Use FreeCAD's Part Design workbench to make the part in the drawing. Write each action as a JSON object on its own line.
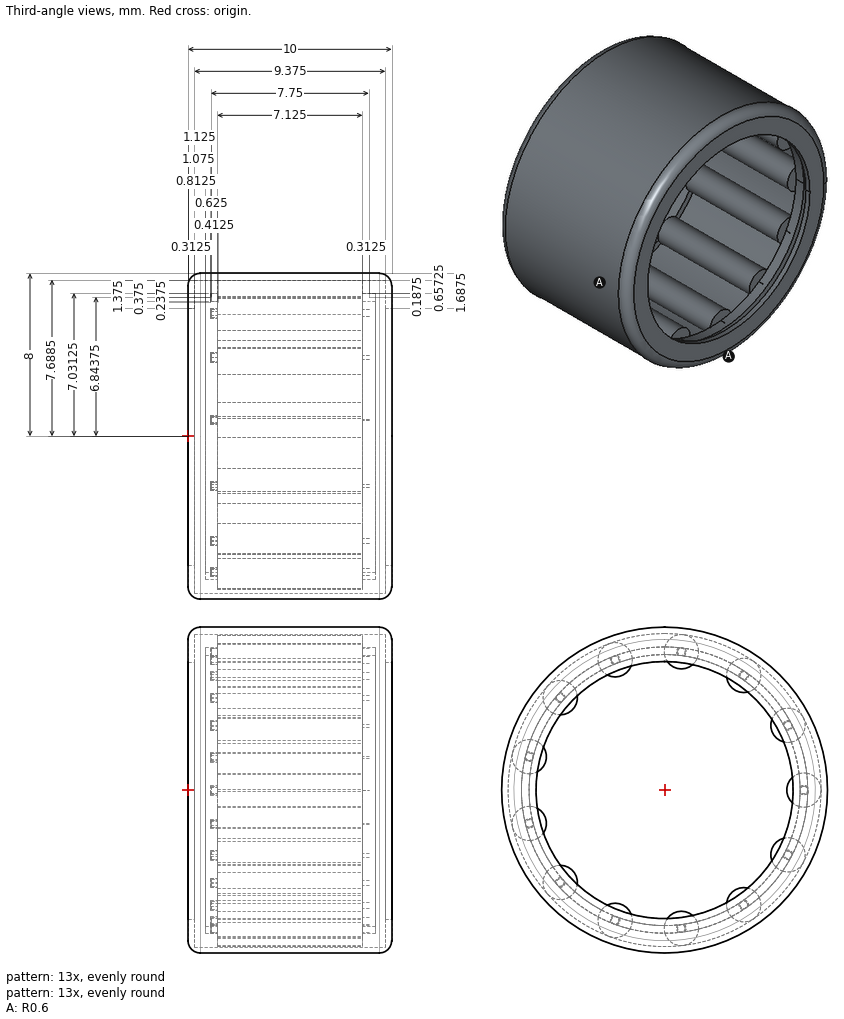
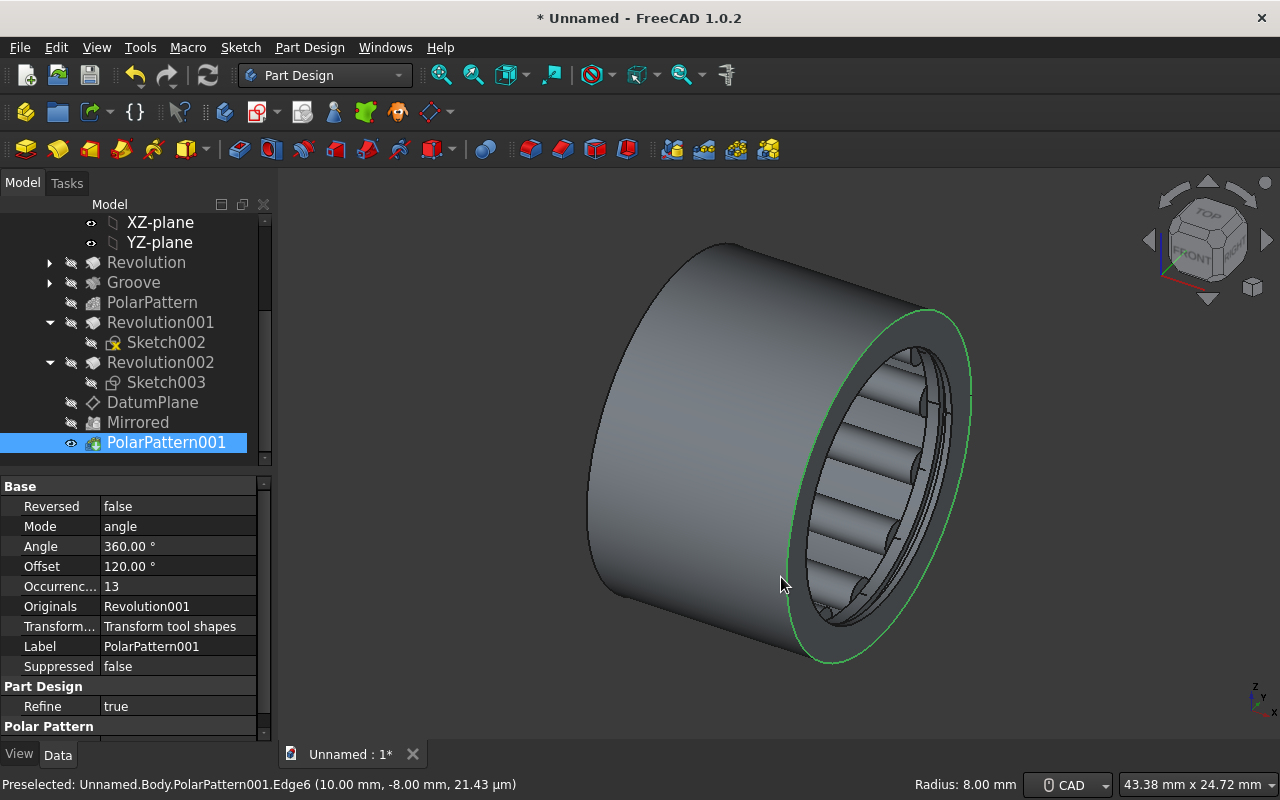
{"action": "key", "text": "0"}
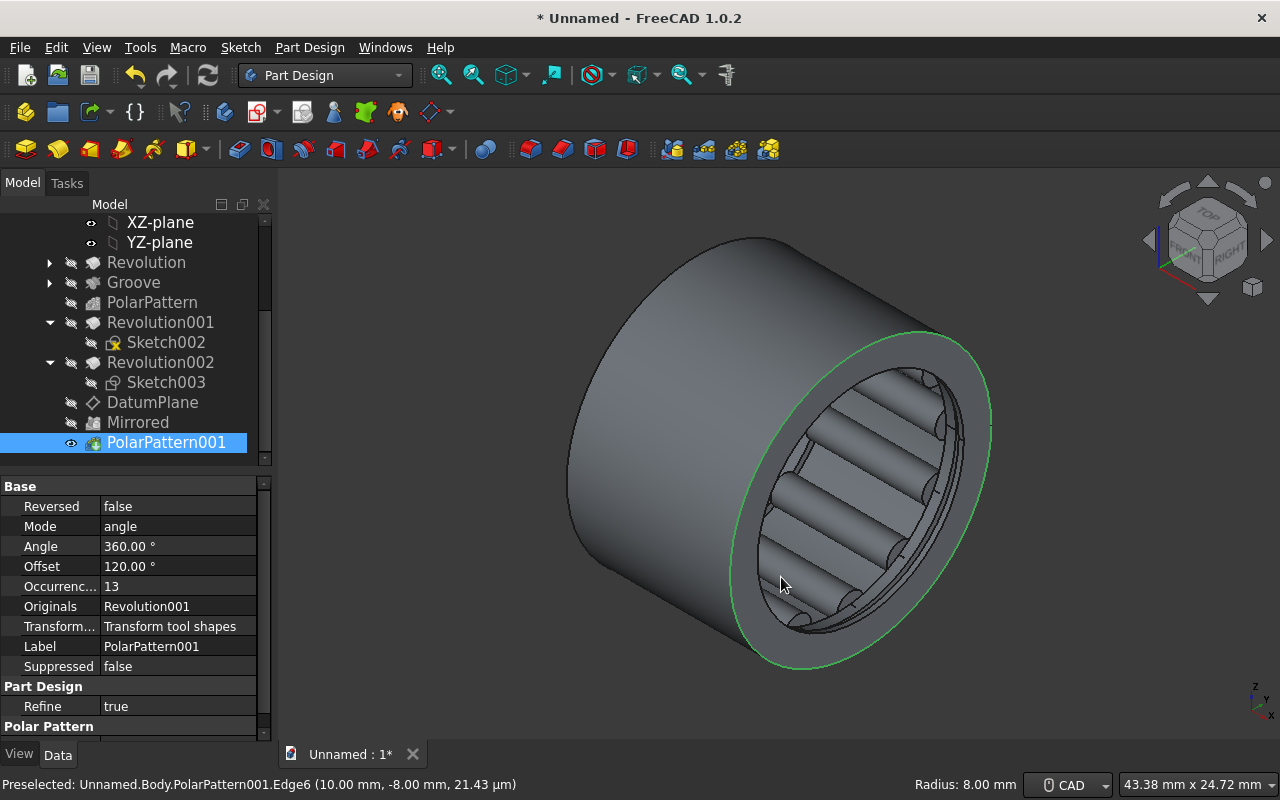
{"action": "key", "text": "2"}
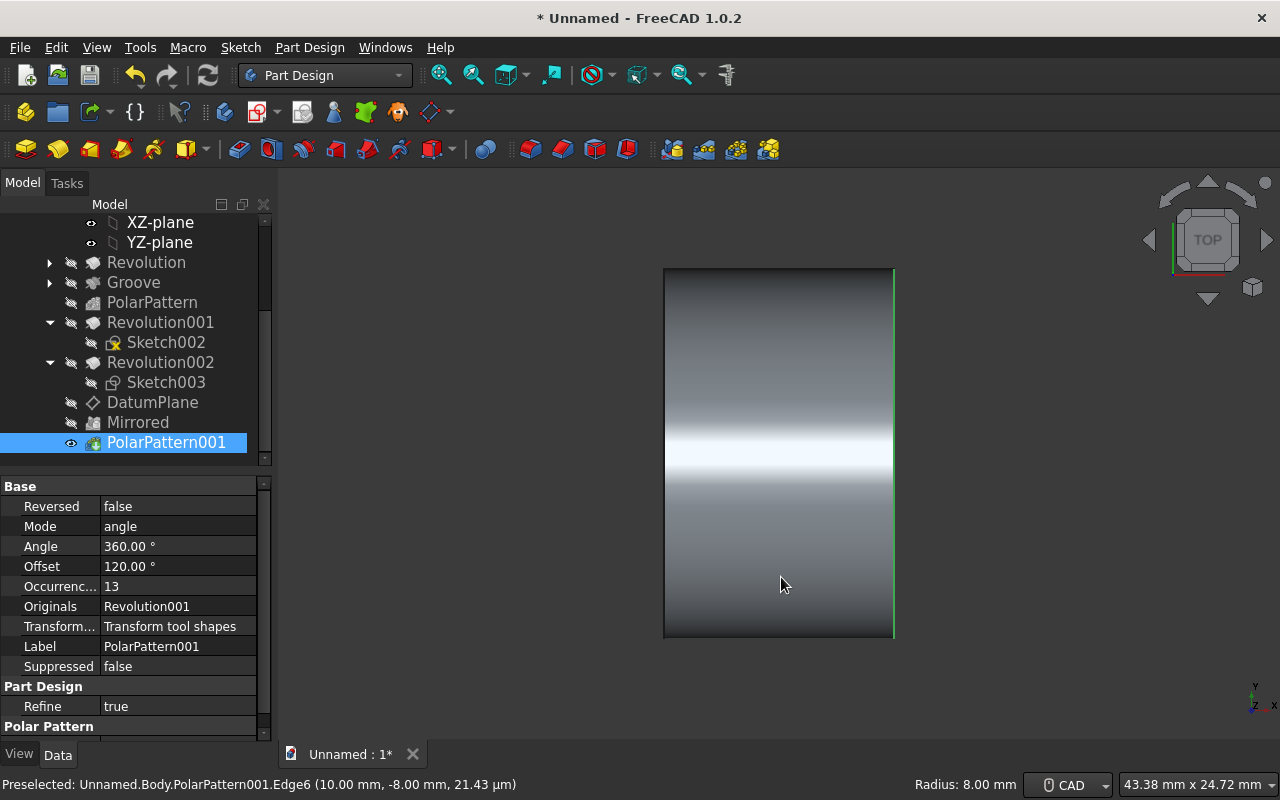
{"action": "left_click", "coordinate": [664, 602], "text": "ctrl"}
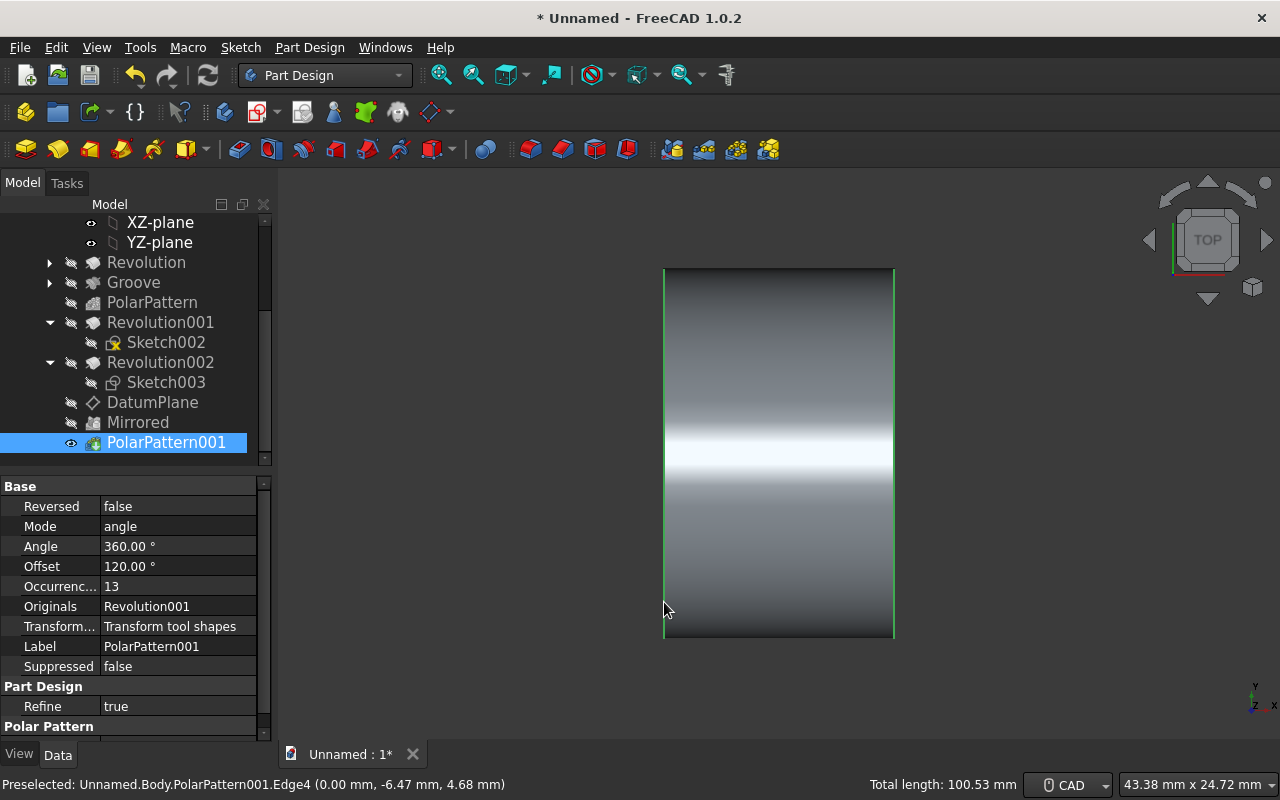
{"action": "left_click", "coordinate": [532, 150]}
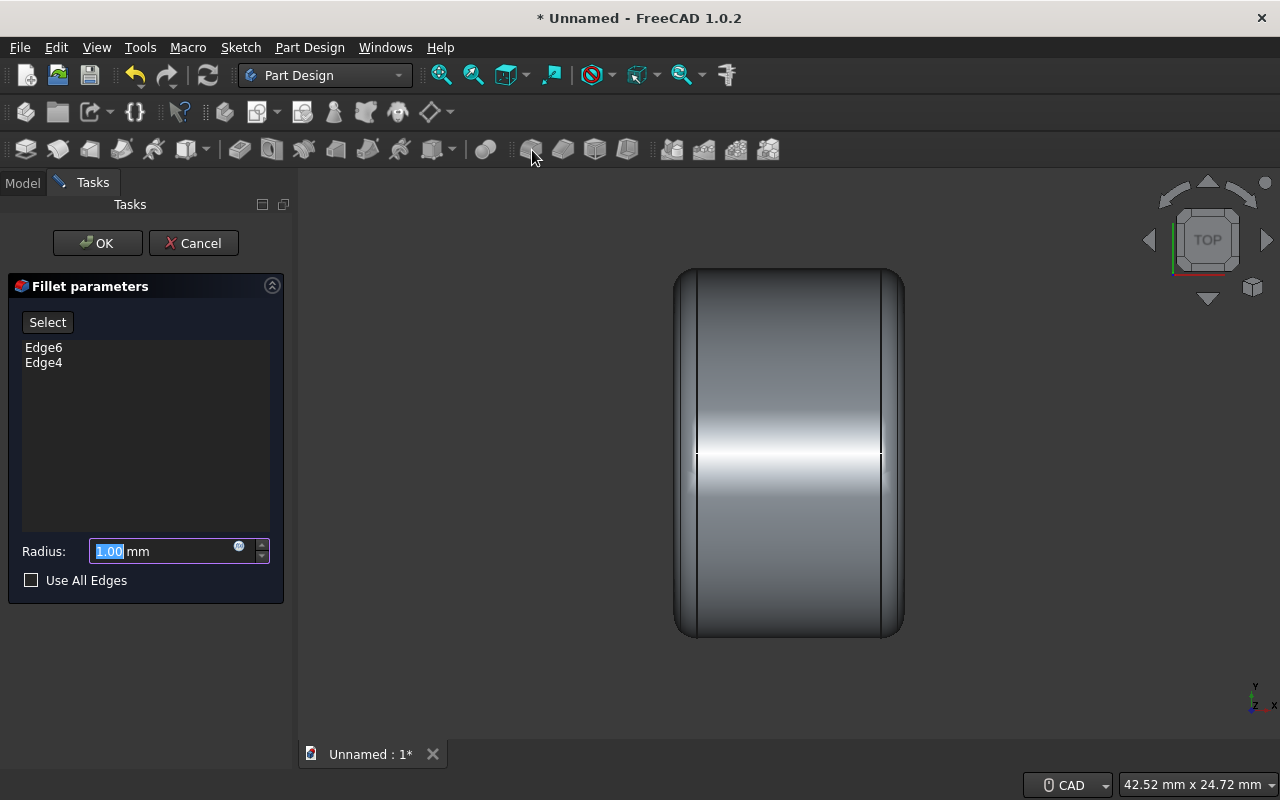
{"action": "type", "text": "0.6"}
{"action": "key", "text": "Tab"}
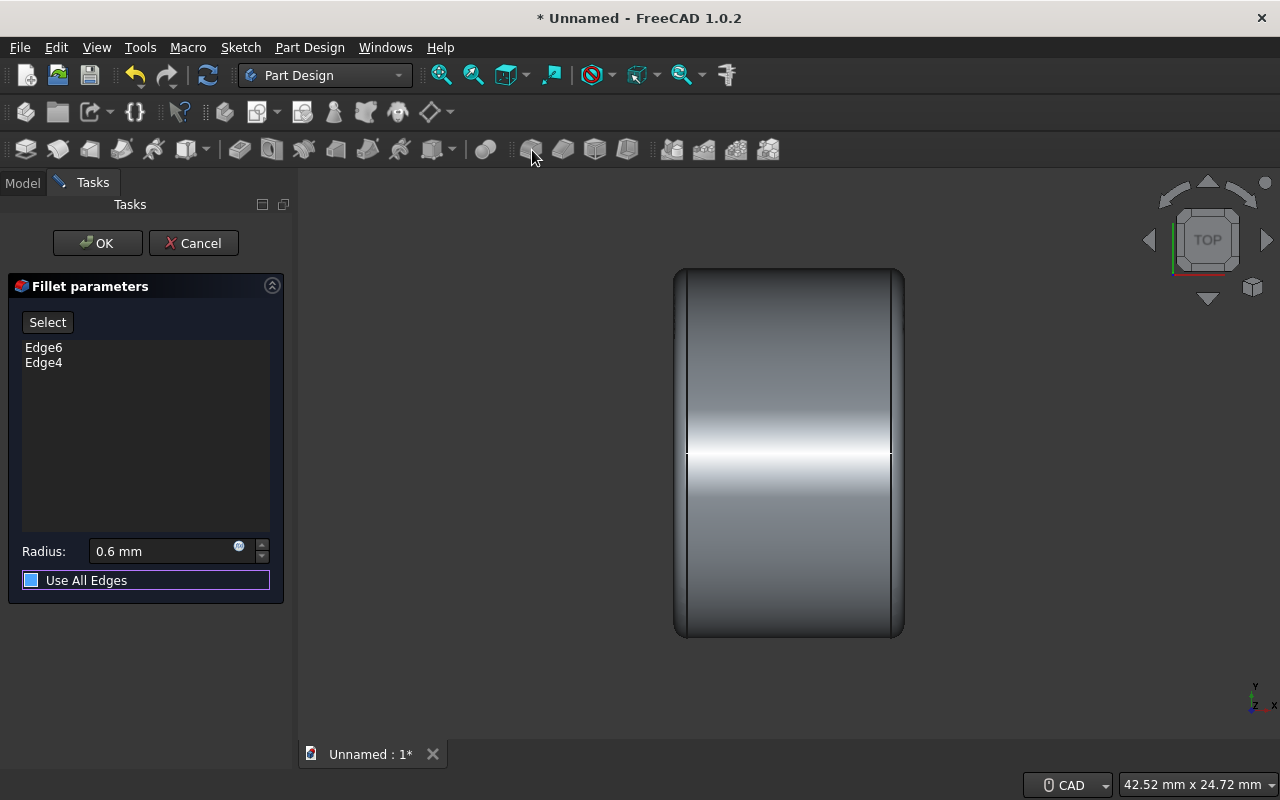
{"action": "left_click", "coordinate": [98, 243]}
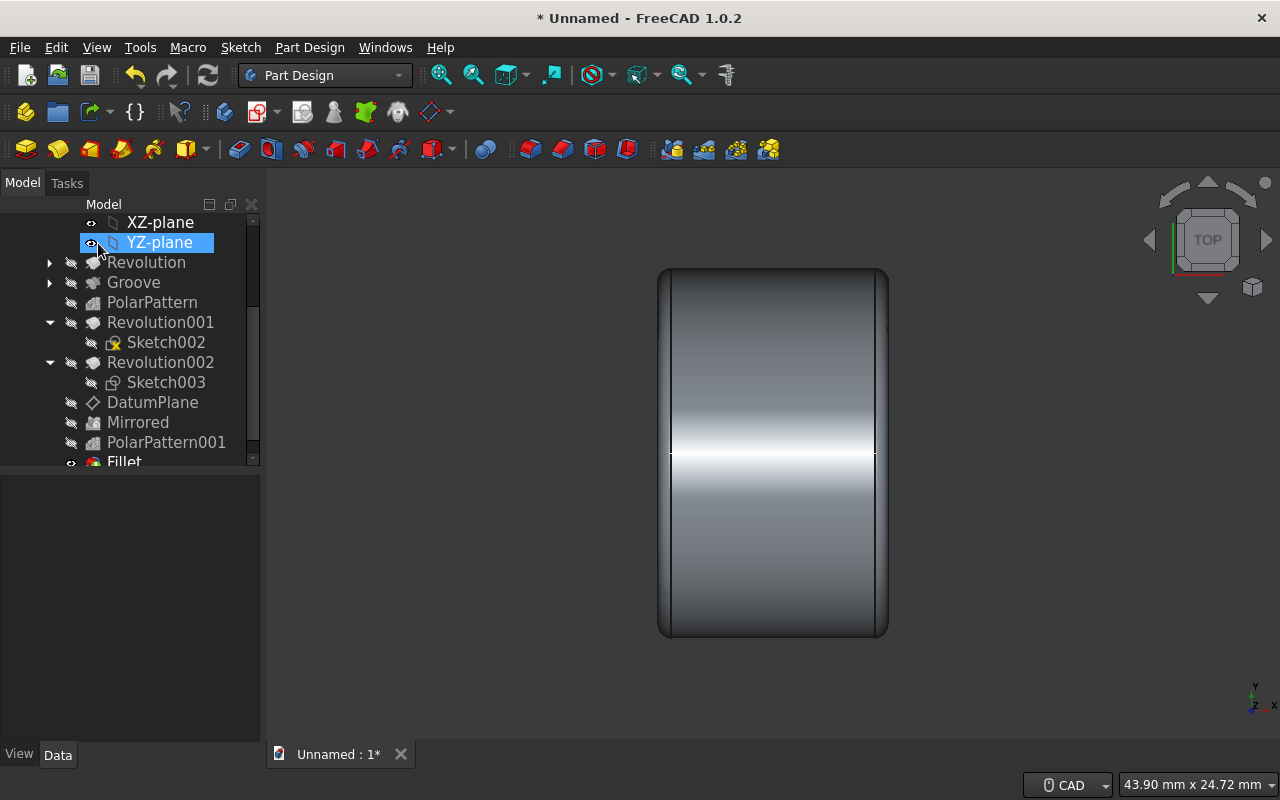
{"action": "scroll", "coordinate": [160, 338], "scroll_direction": "down", "scroll_amount": 3}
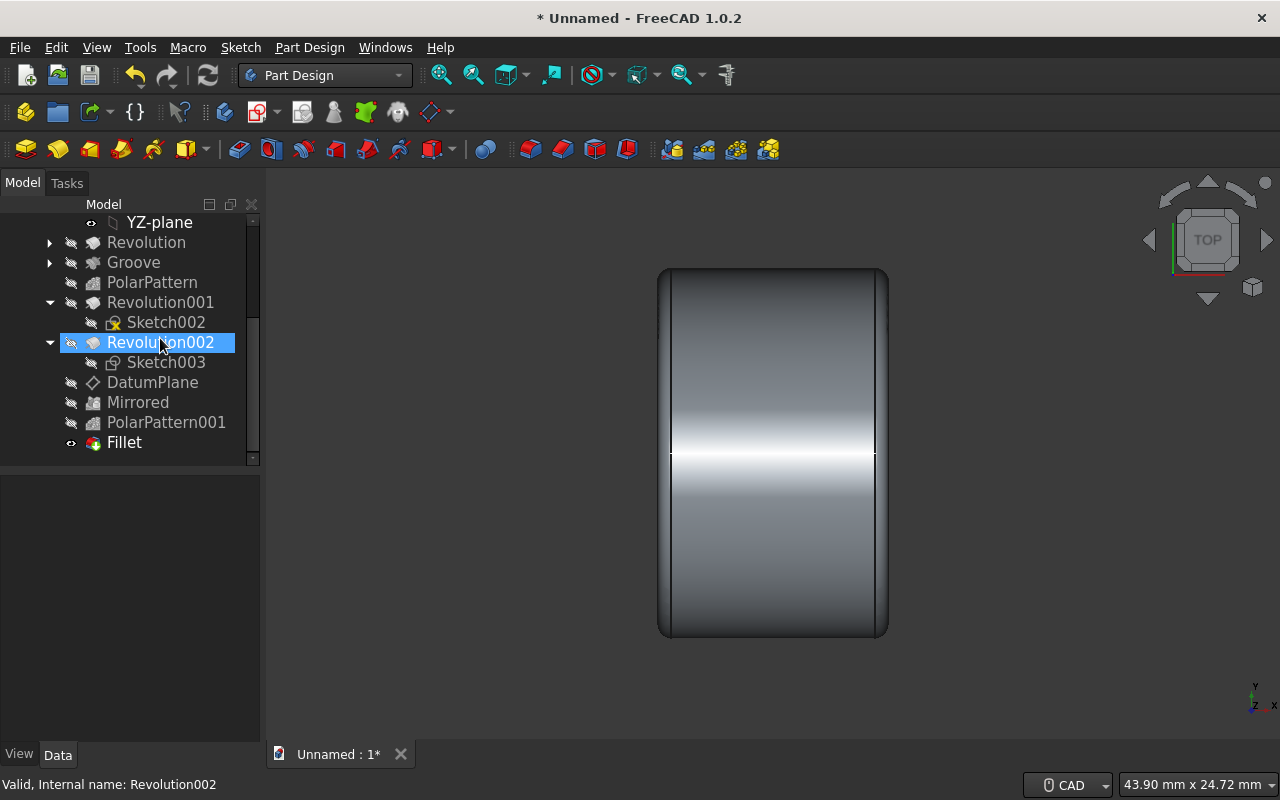
{"action": "scroll", "coordinate": [160, 338], "scroll_direction": "up", "scroll_amount": 15}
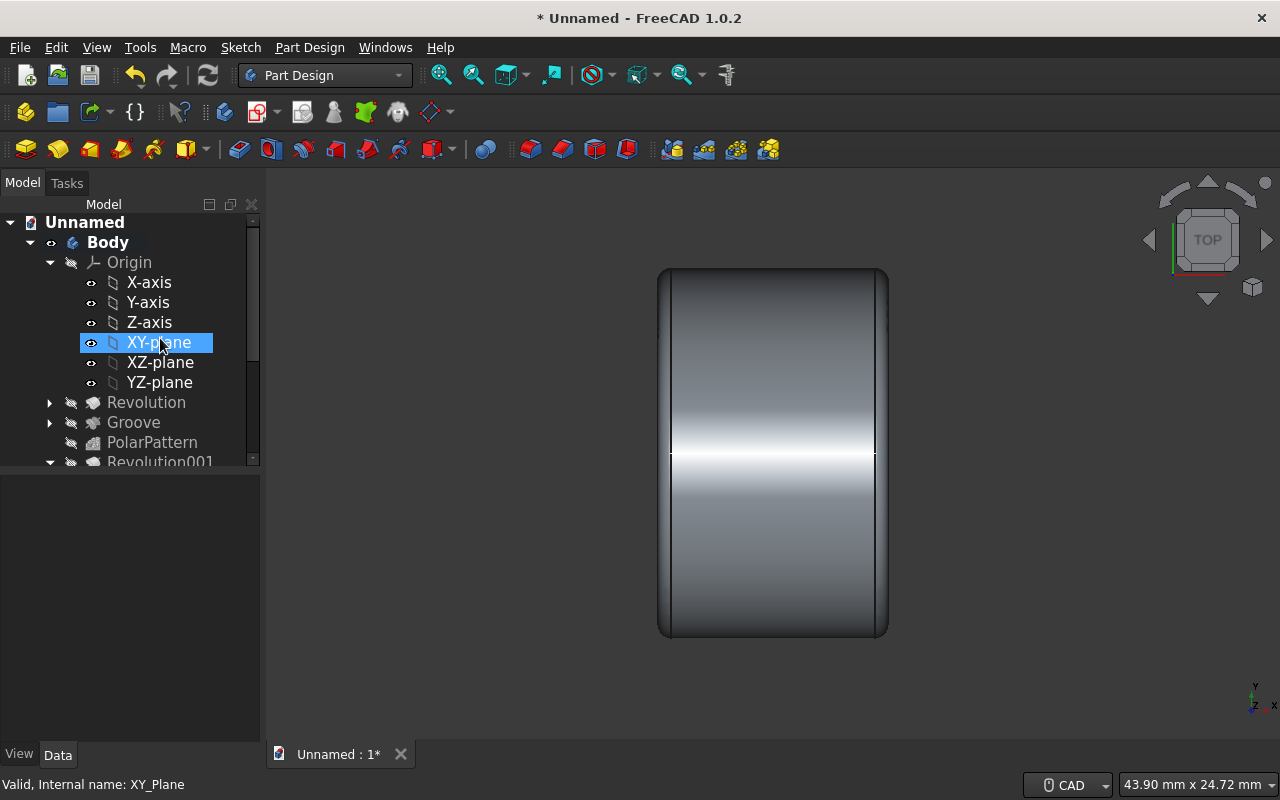
{"action": "left_click", "coordinate": [136, 383]}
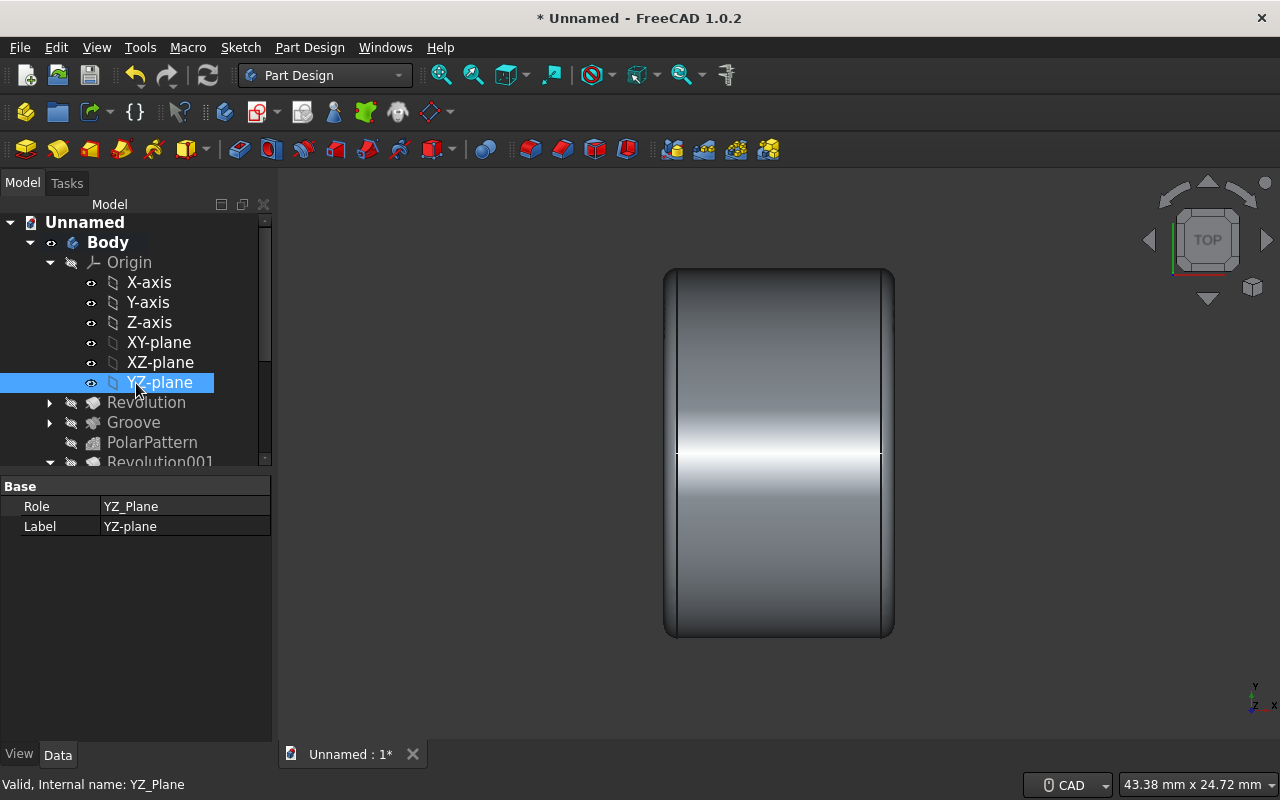
{"action": "left_click", "coordinate": [430, 112]}